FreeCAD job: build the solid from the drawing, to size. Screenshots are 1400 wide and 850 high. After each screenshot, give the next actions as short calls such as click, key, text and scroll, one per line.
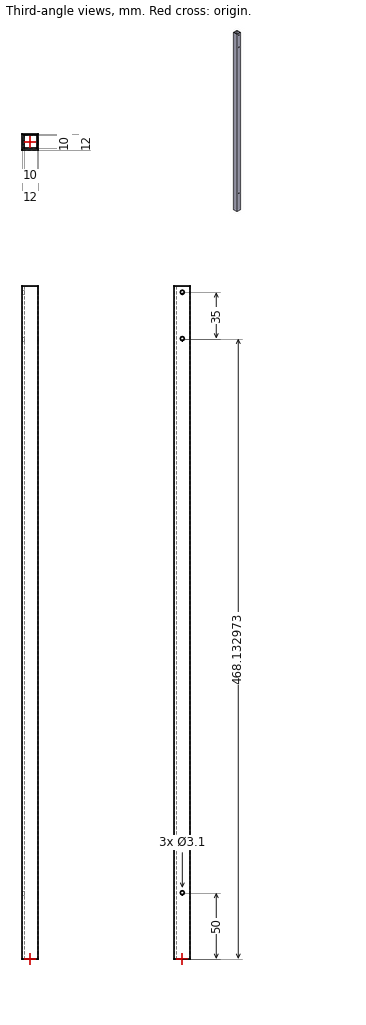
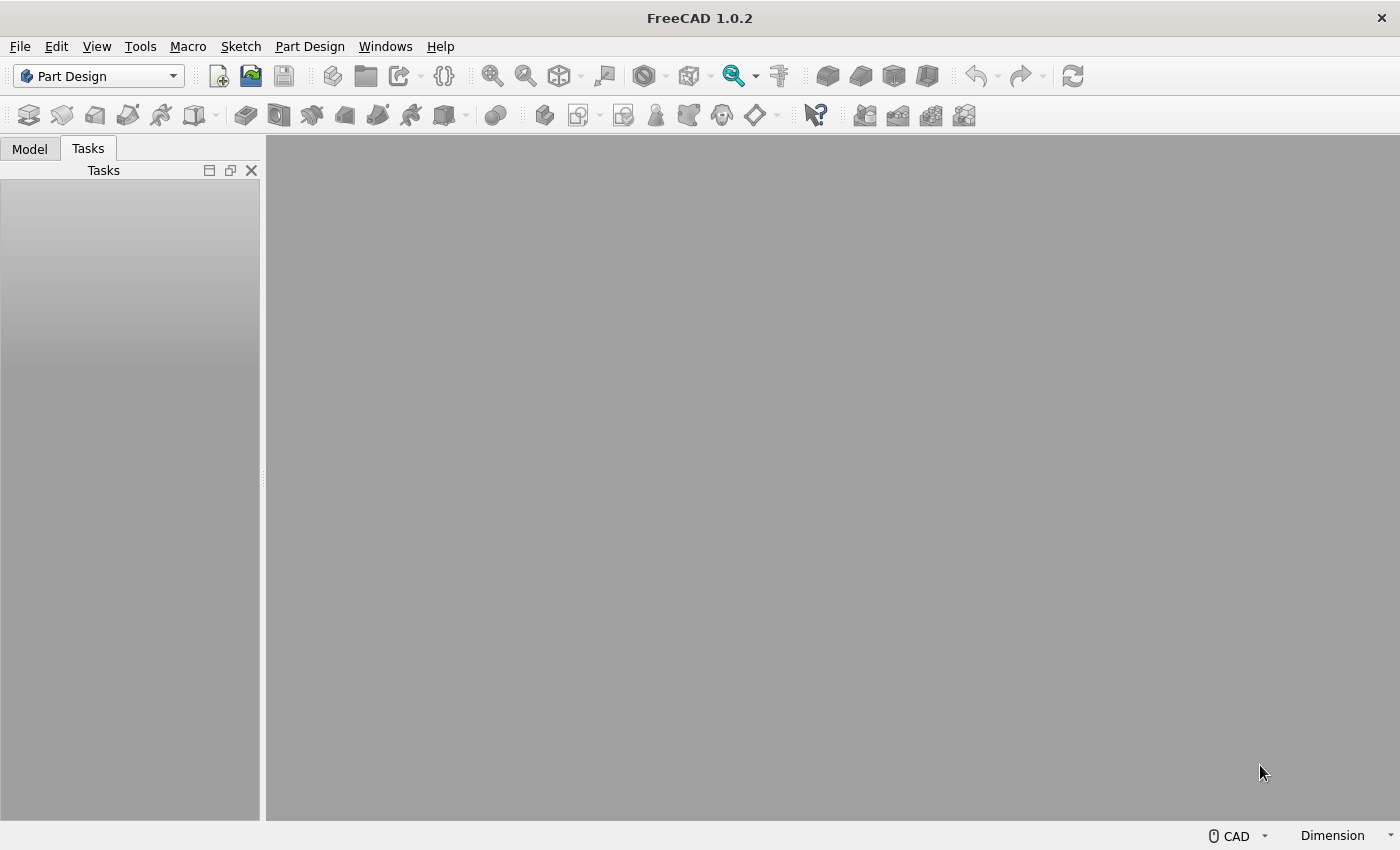
click(218, 76)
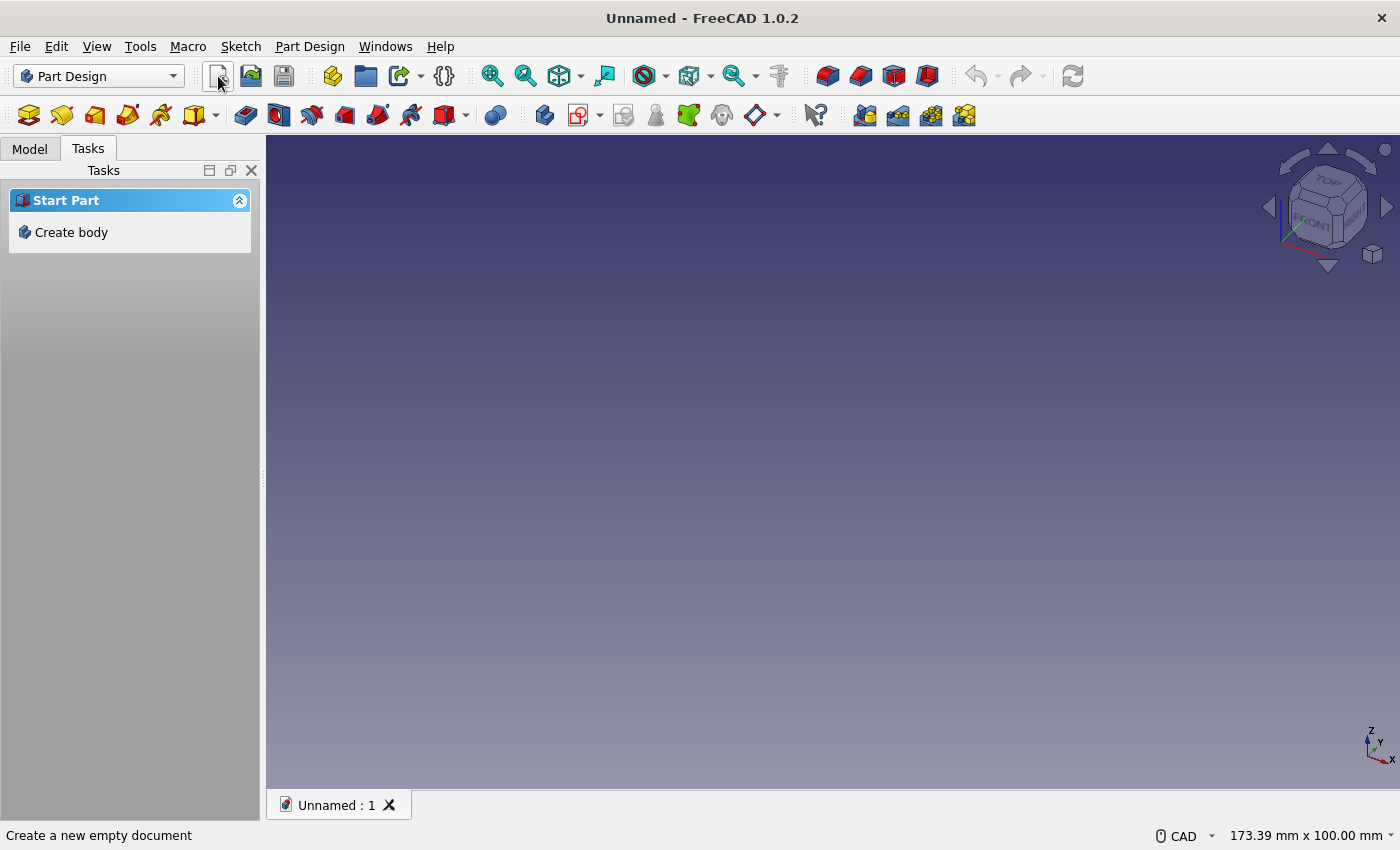
click(578, 116)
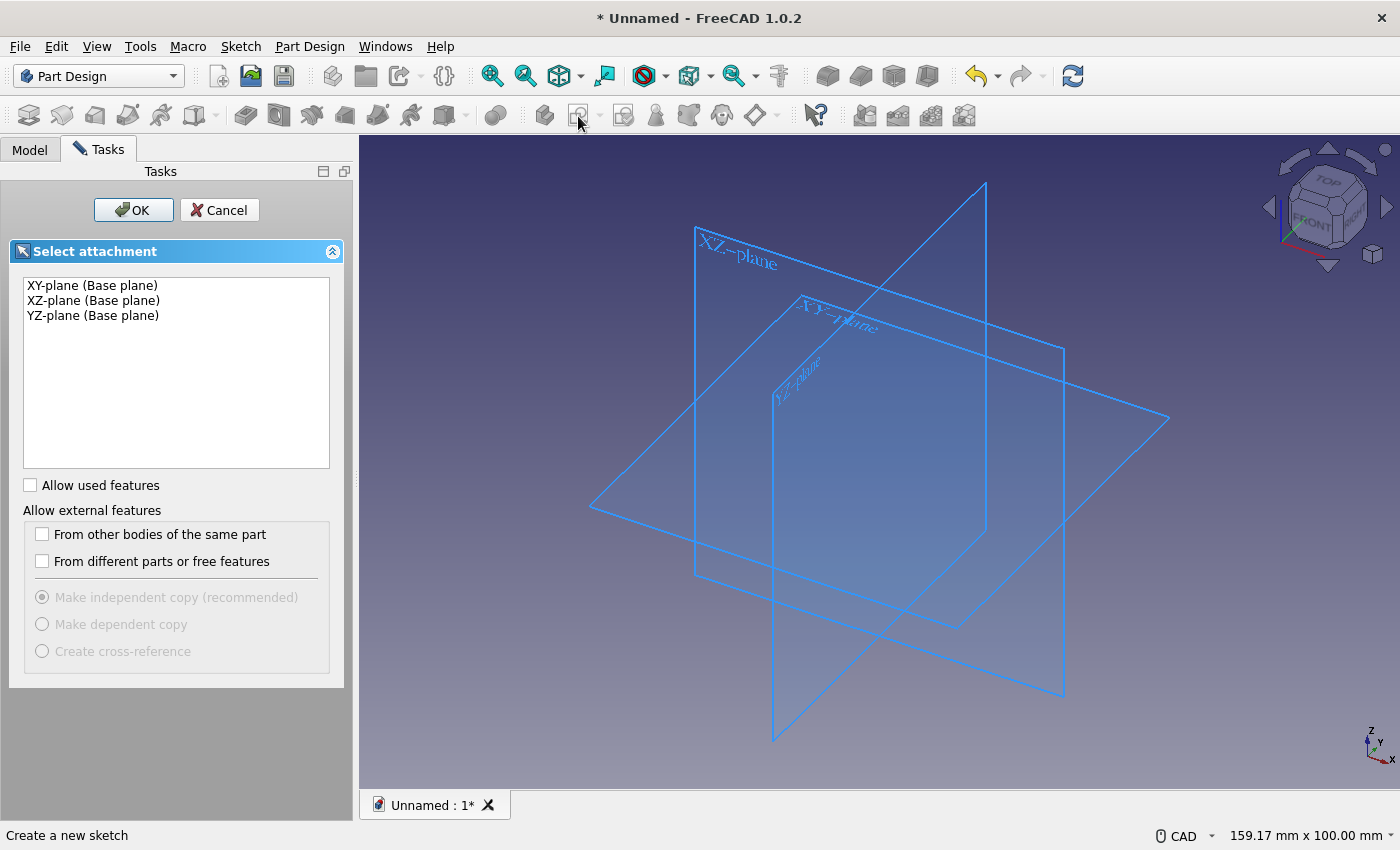
click(84, 286)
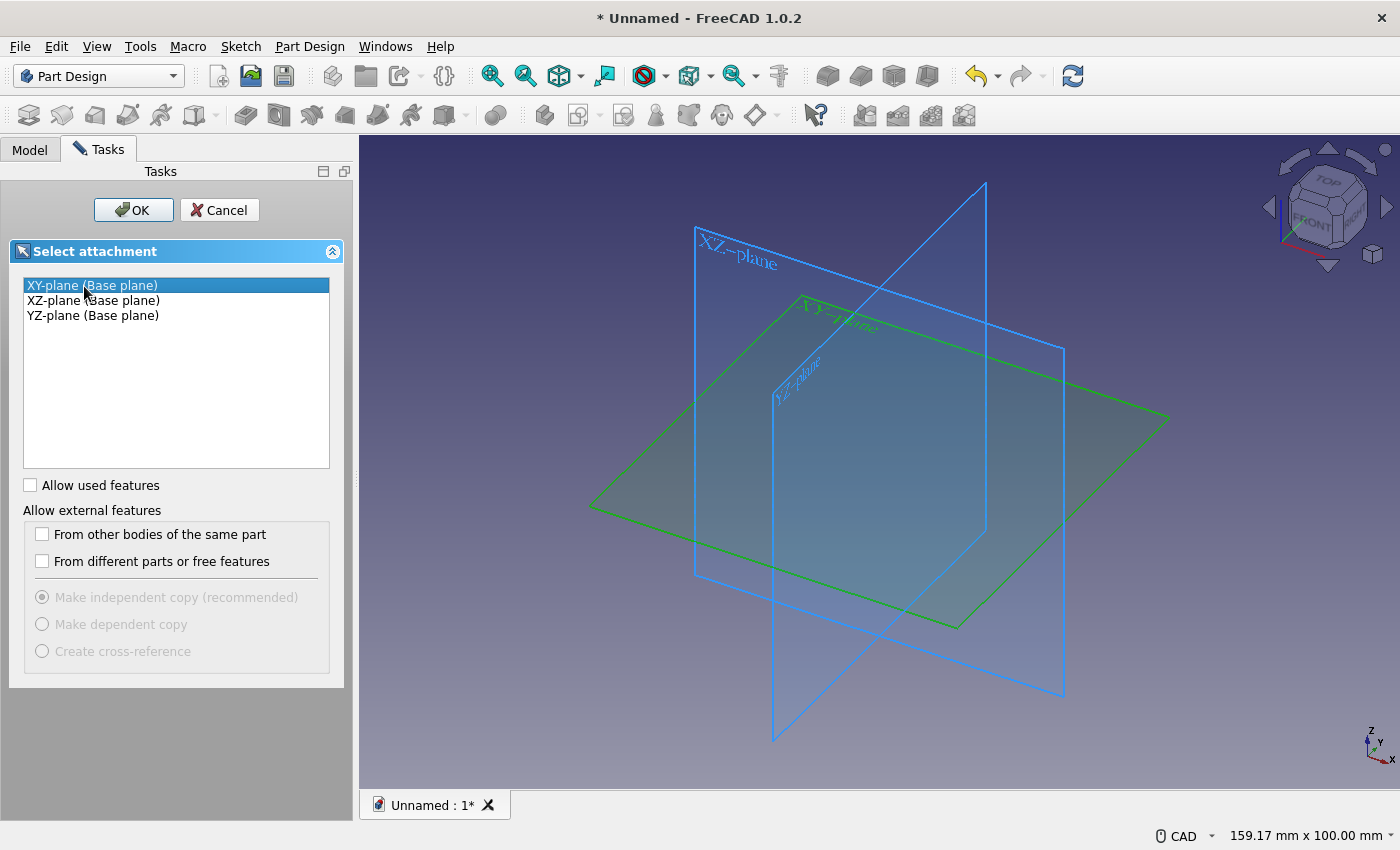
click(134, 210)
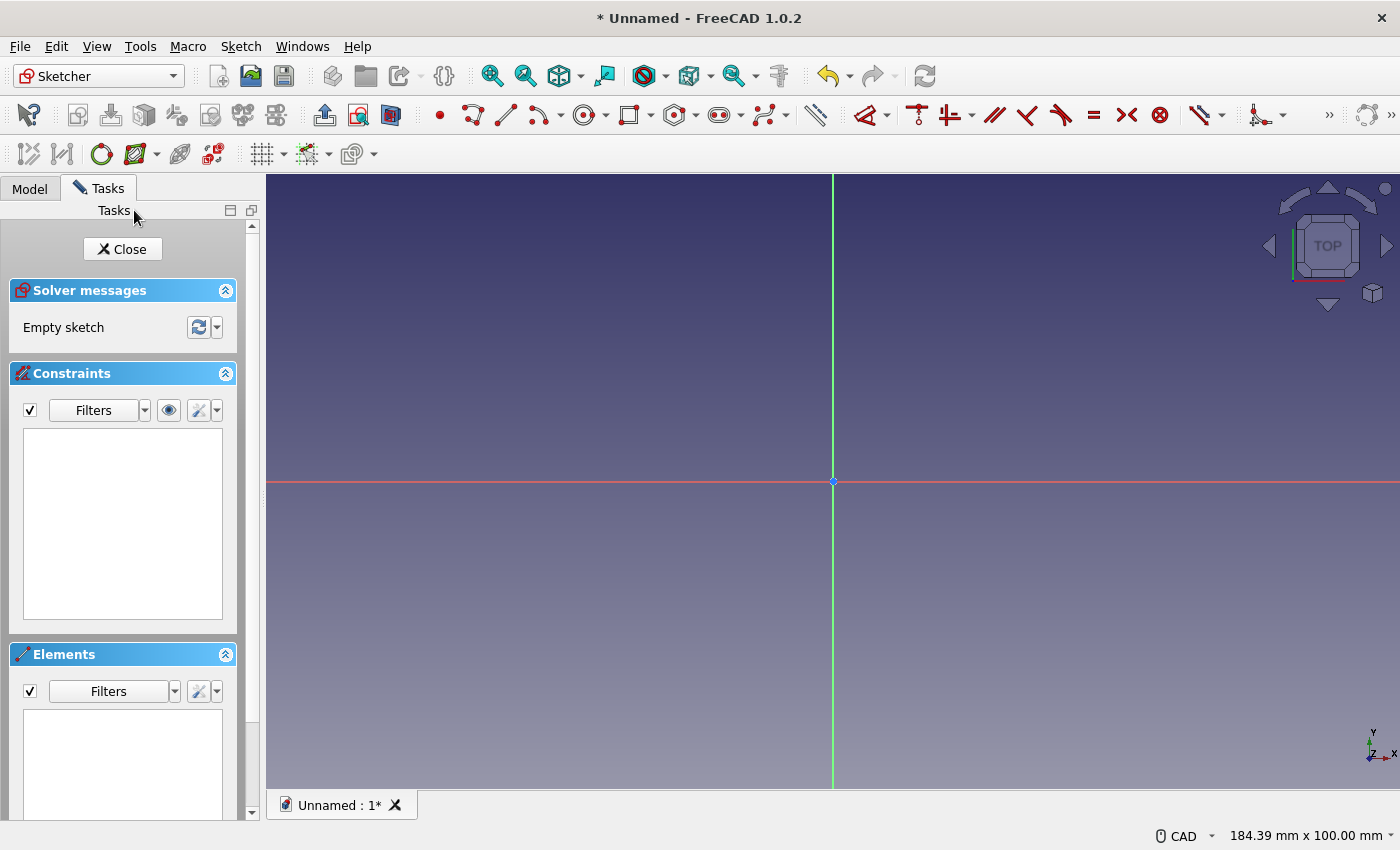
scroll(850, 482, up, 8)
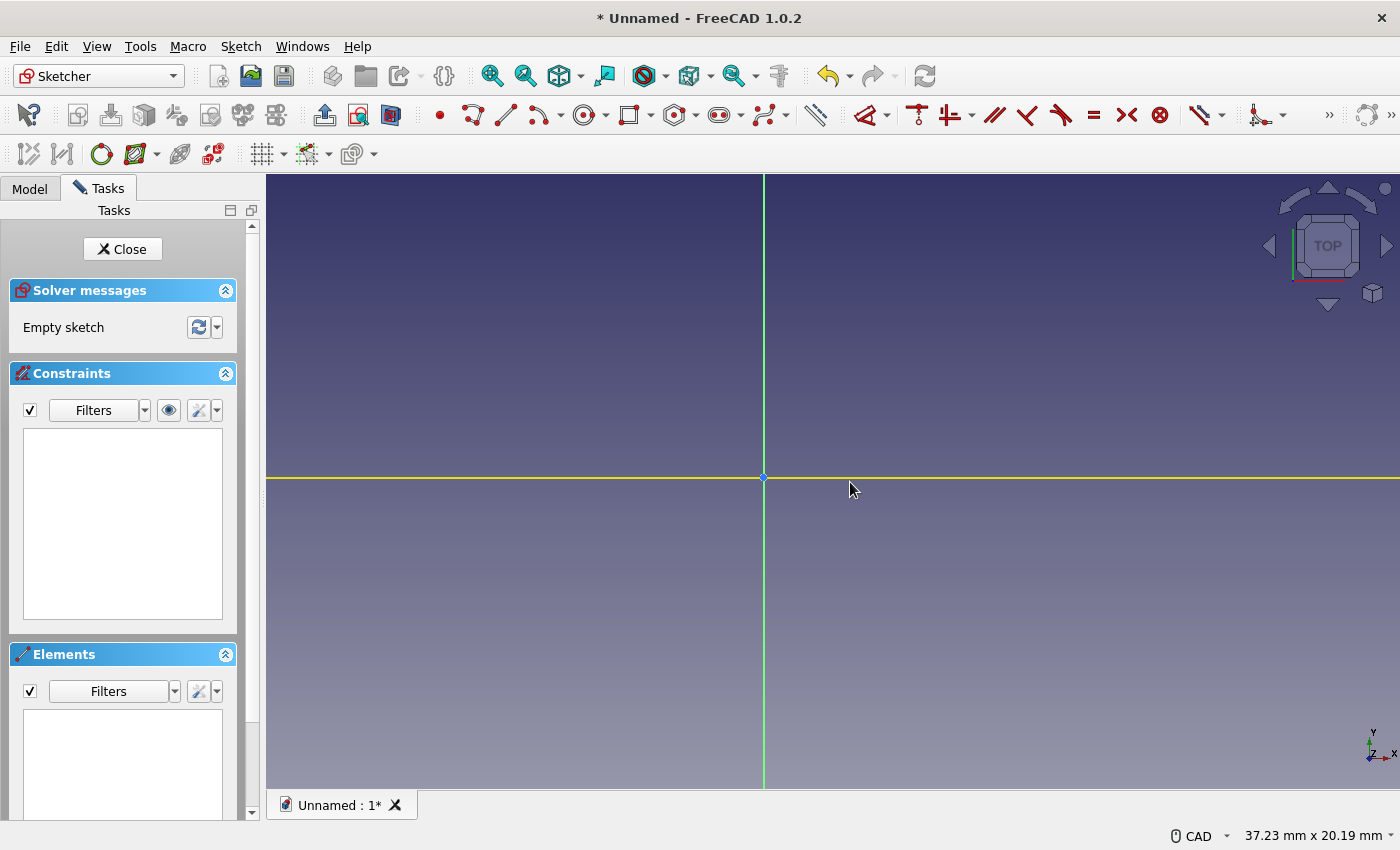
key(g)
key(v)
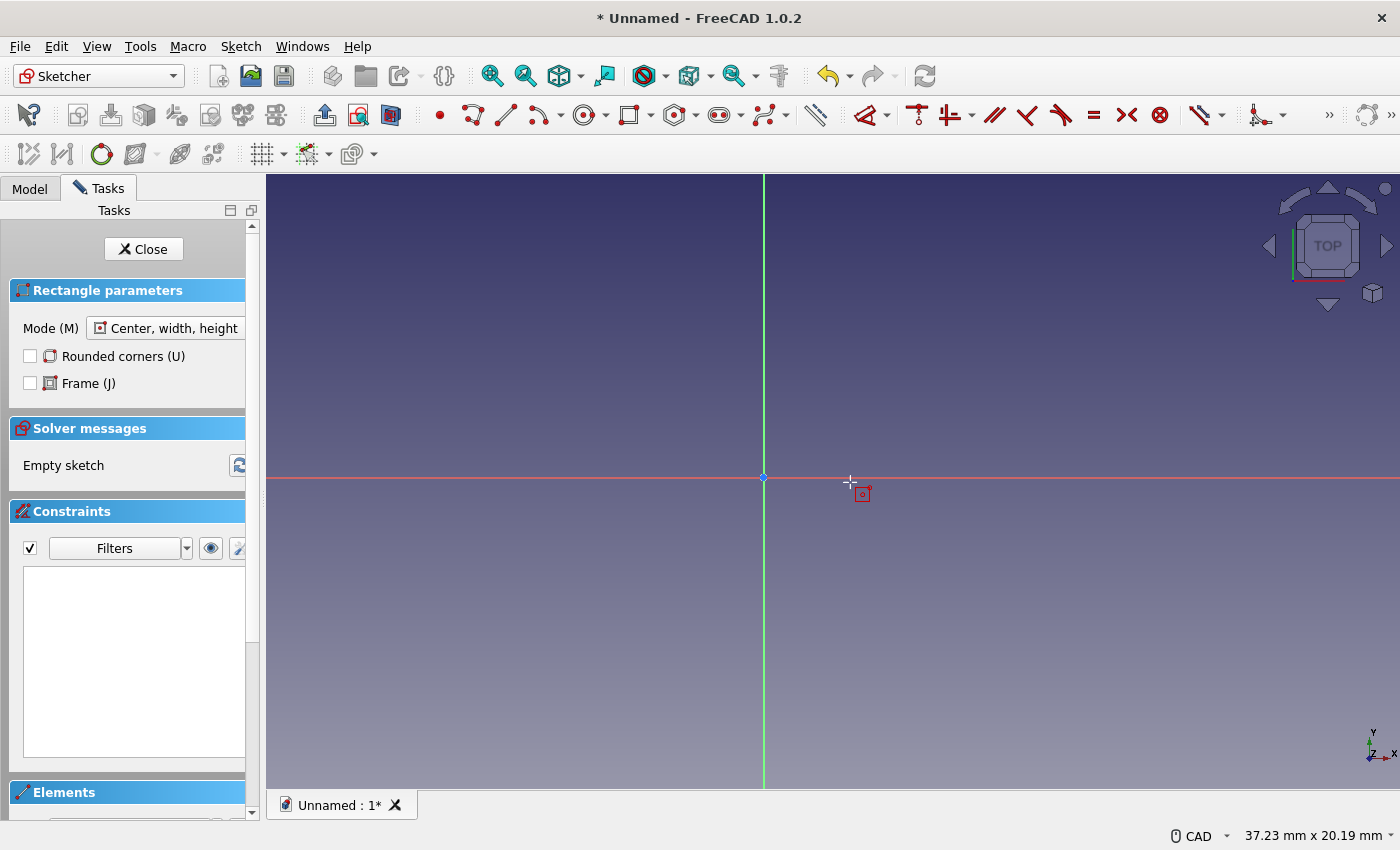
click(764, 478)
click(947, 295)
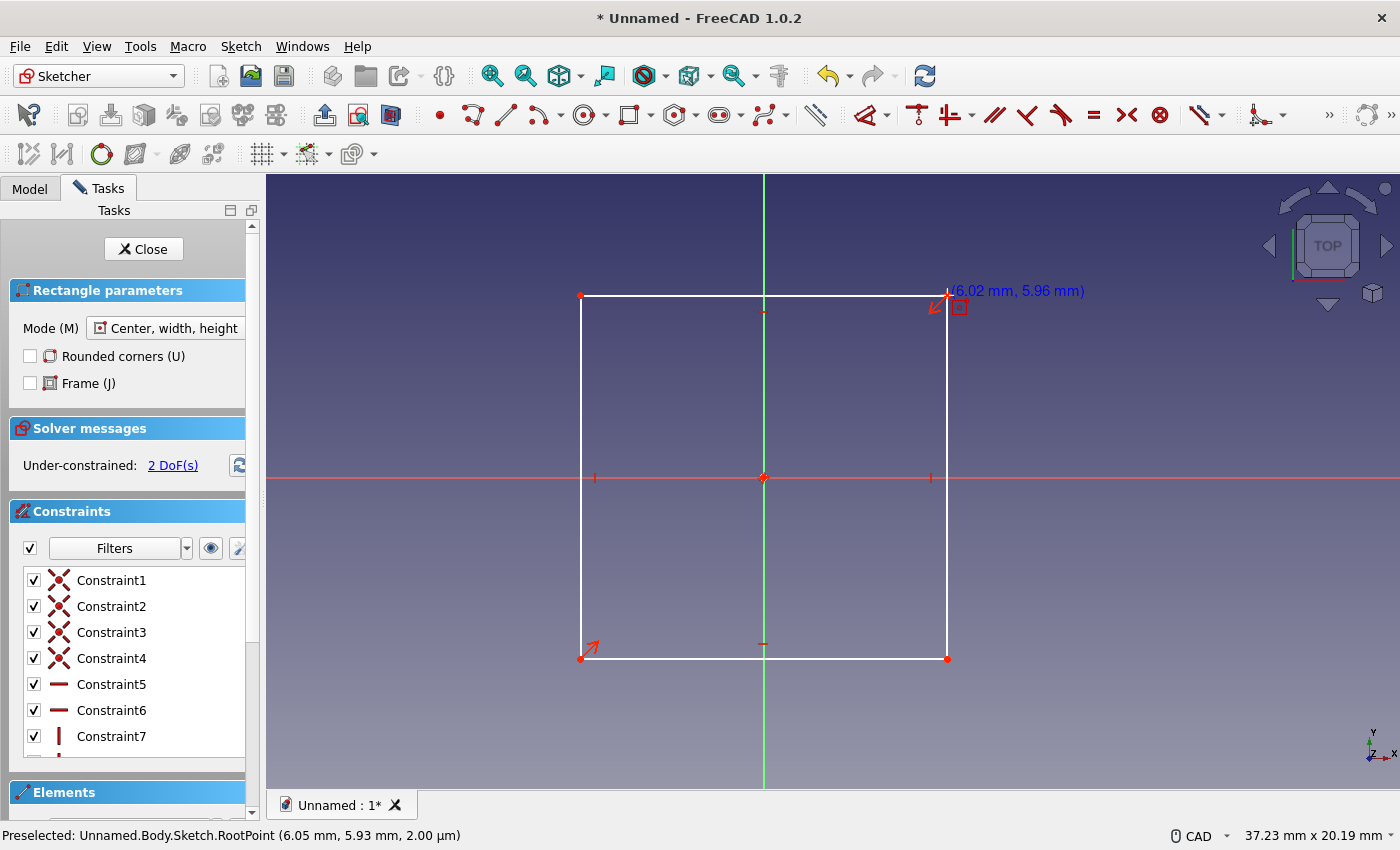
click(764, 478)
click(916, 325)
key(Escape)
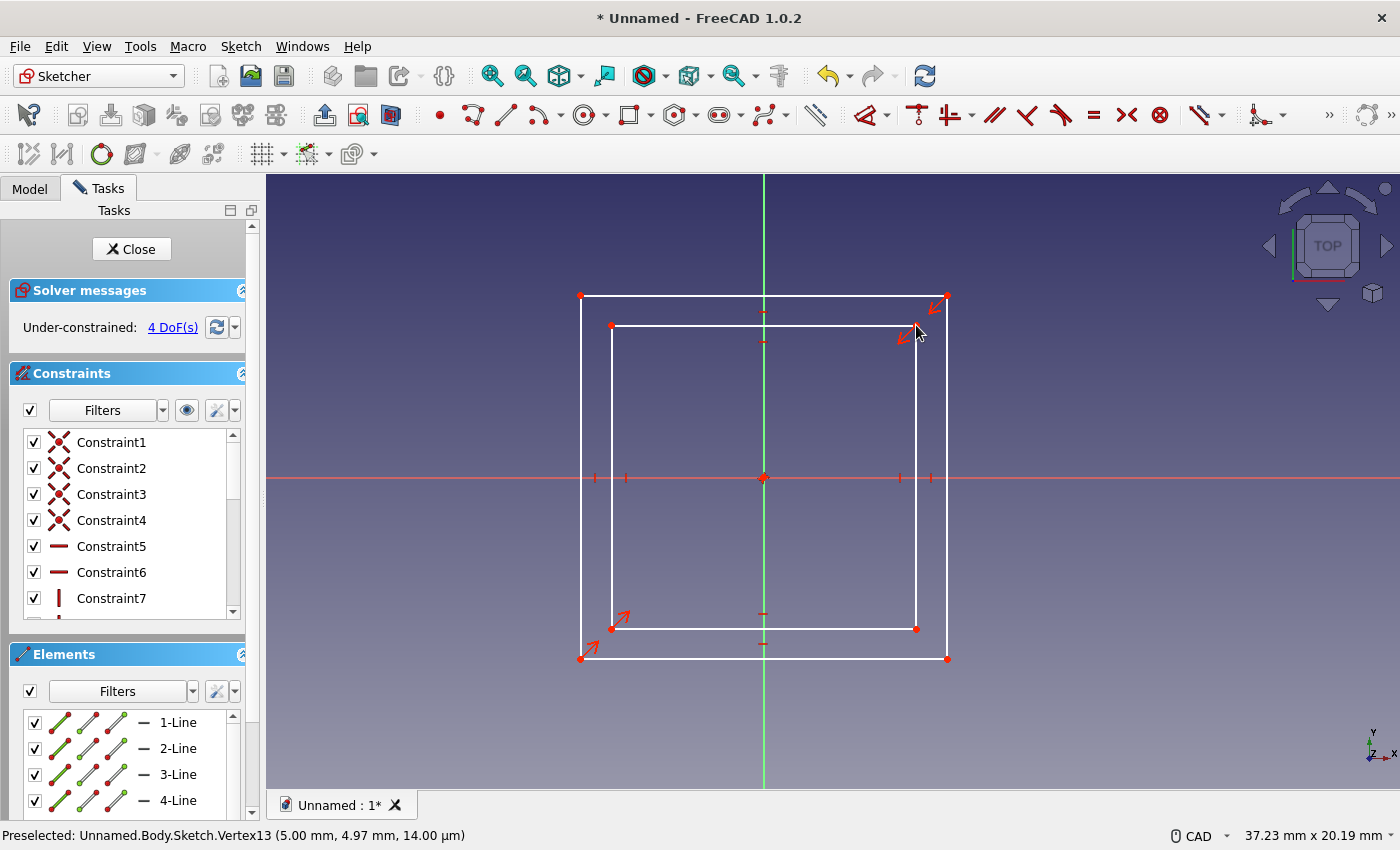
click(690, 659)